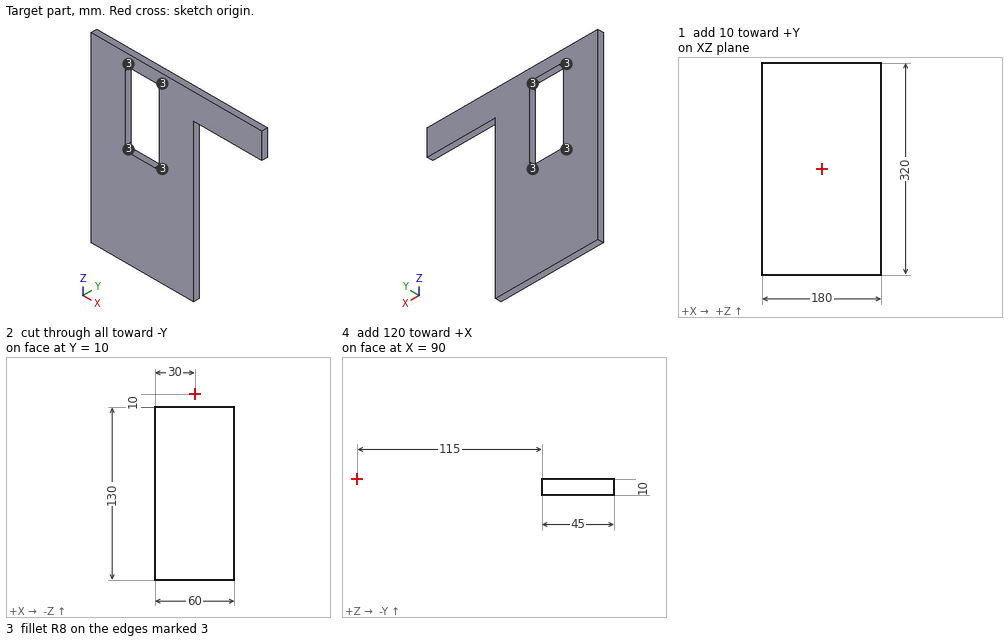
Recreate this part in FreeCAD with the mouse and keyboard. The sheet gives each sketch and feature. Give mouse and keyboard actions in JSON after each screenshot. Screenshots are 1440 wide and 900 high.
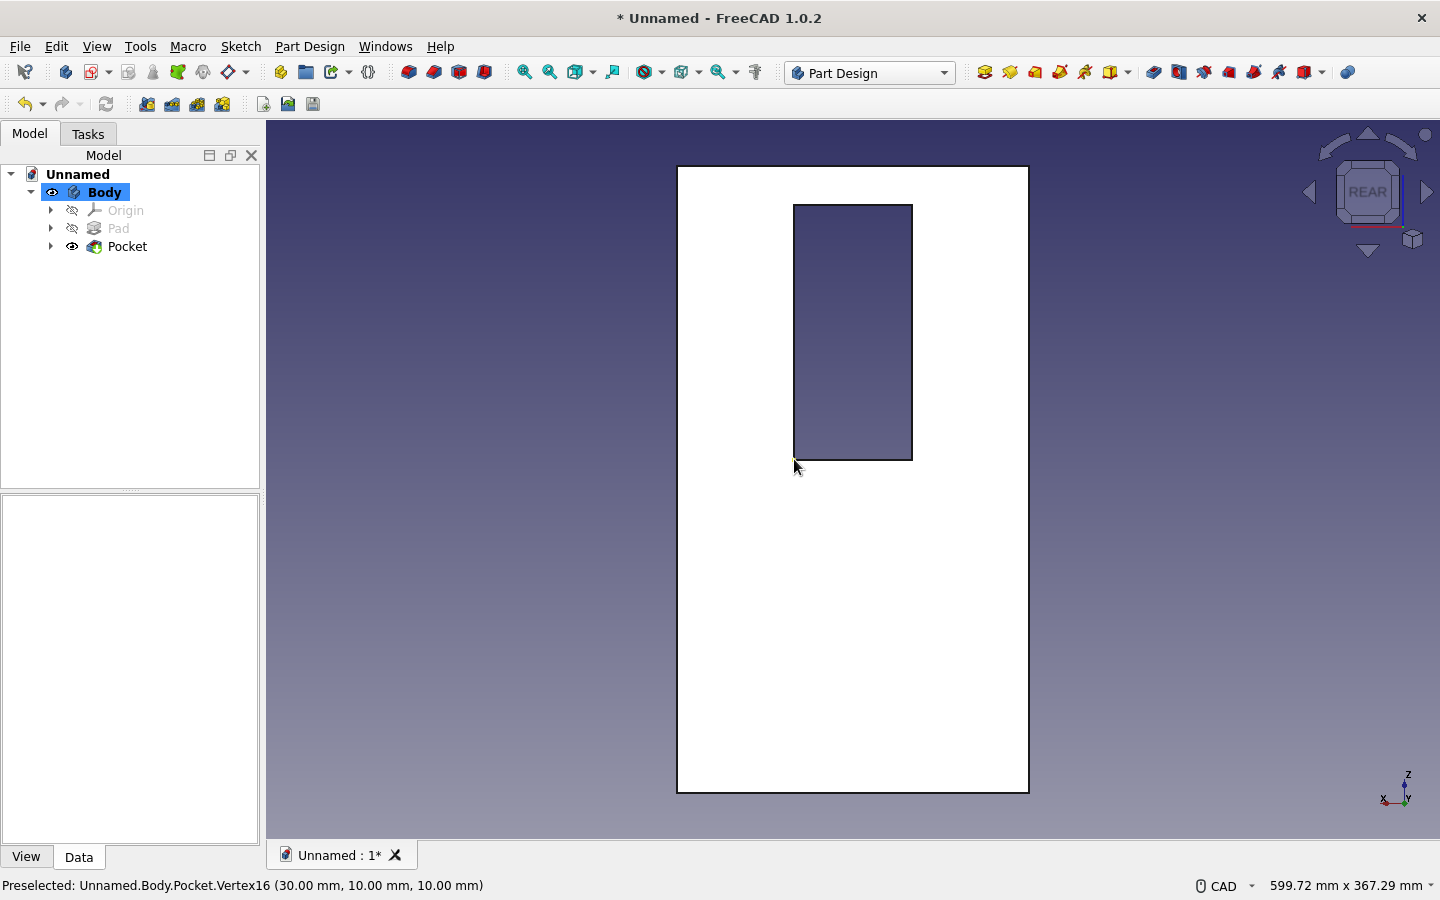
{"action": "key", "text": "0"}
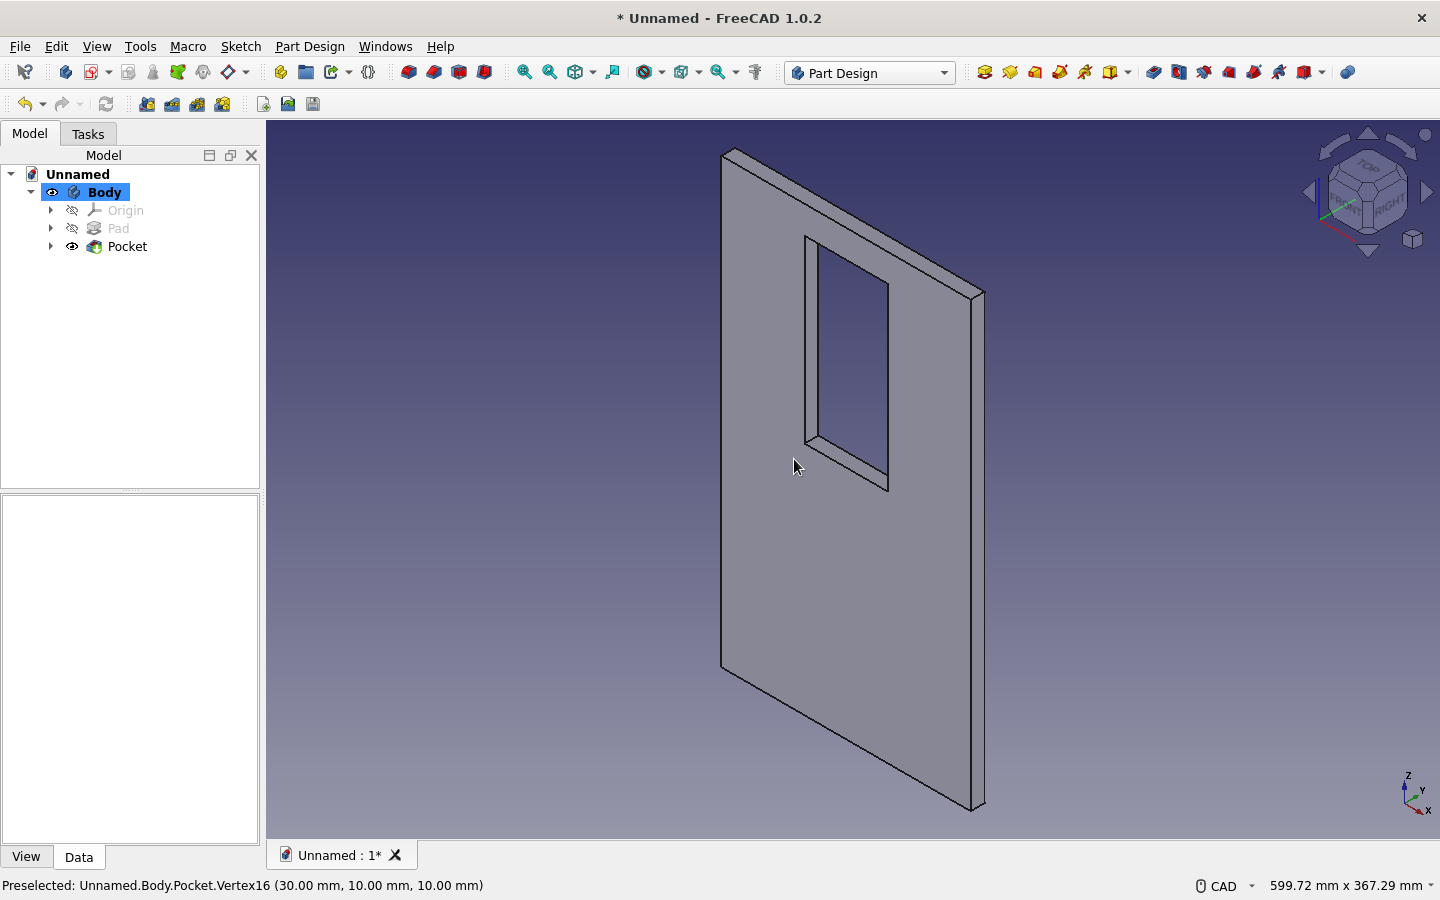
{"action": "scroll", "coordinate": [895, 486], "scroll_direction": "up", "scroll_amount": 4}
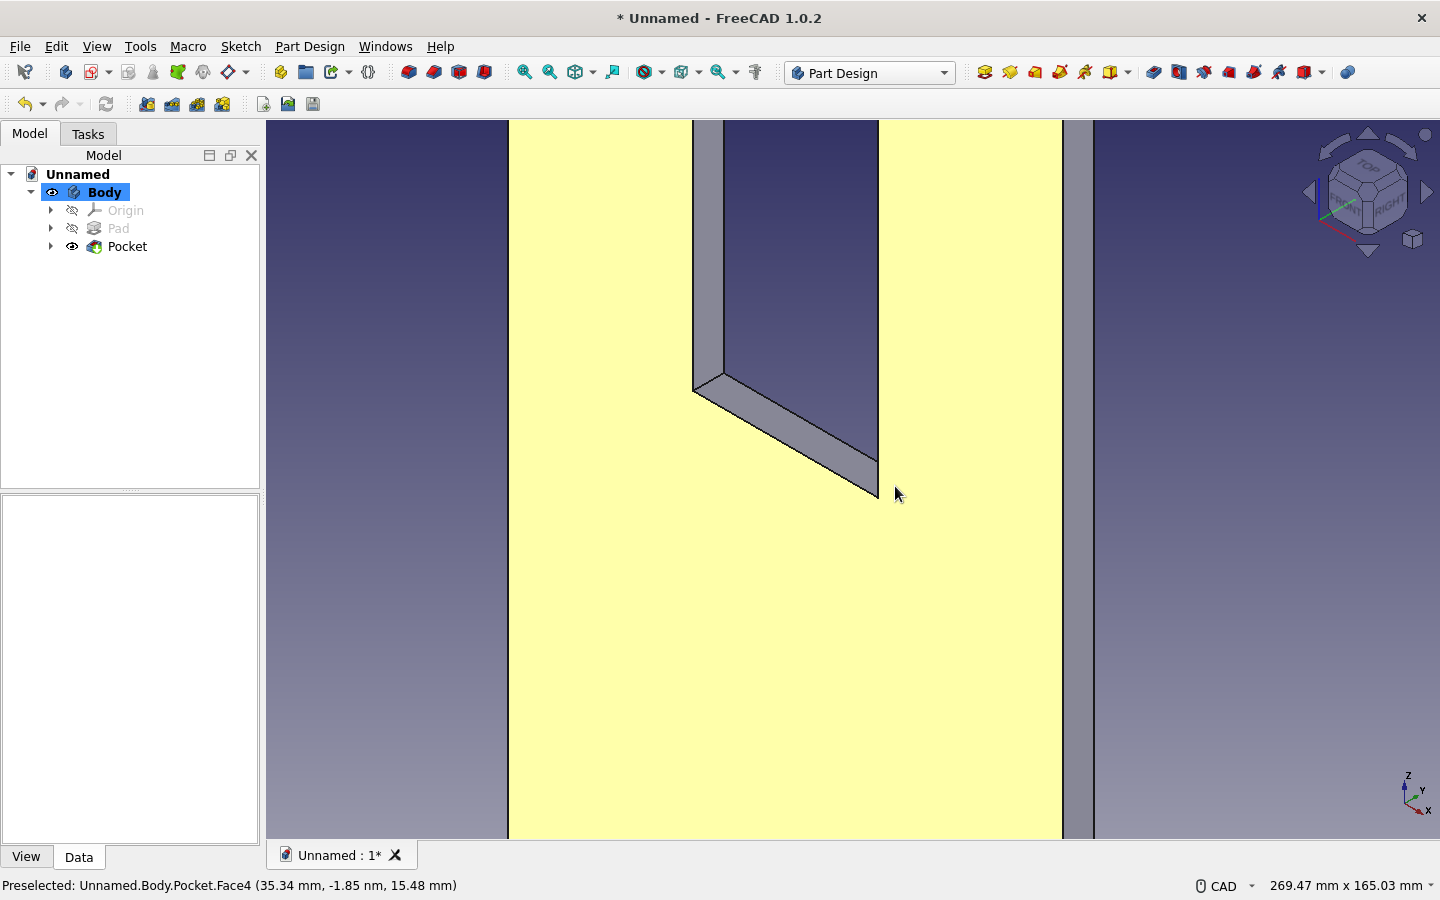
{"action": "key", "text": "v f"}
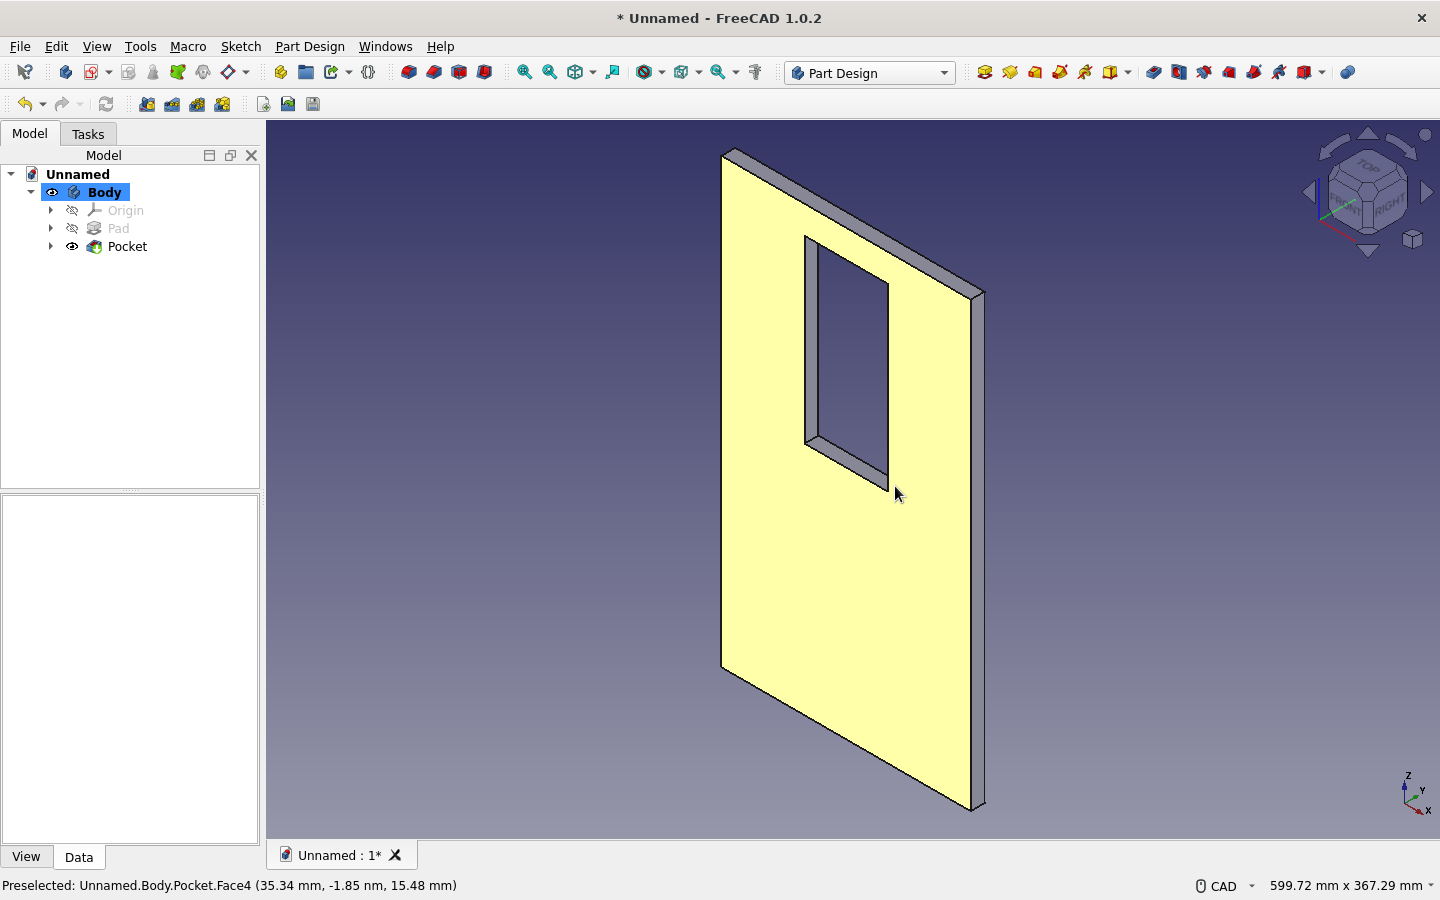
{"action": "key", "text": "2"}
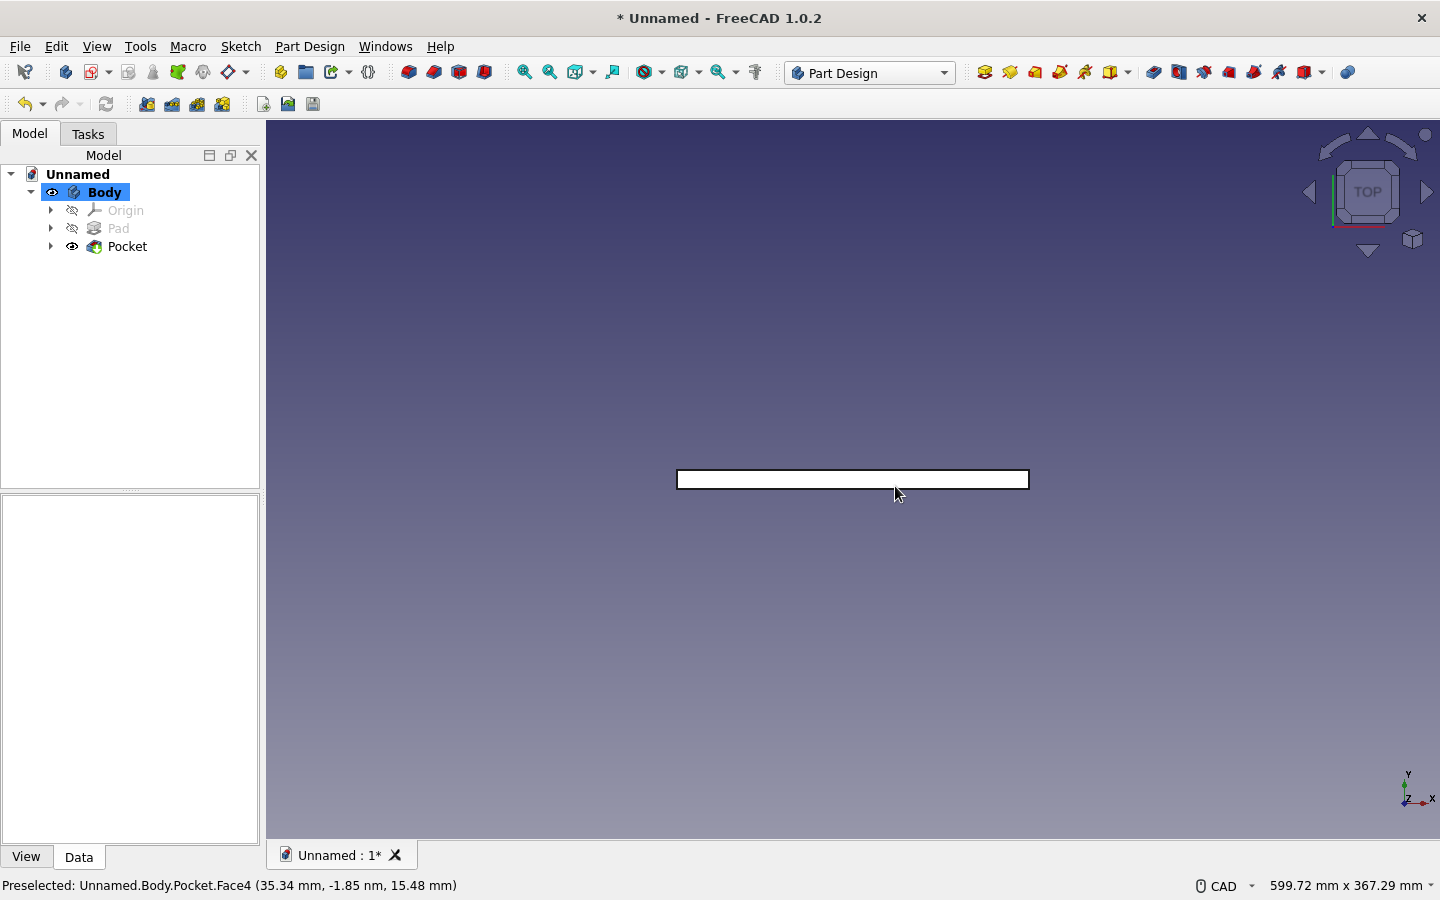
{"action": "key", "text": "v f"}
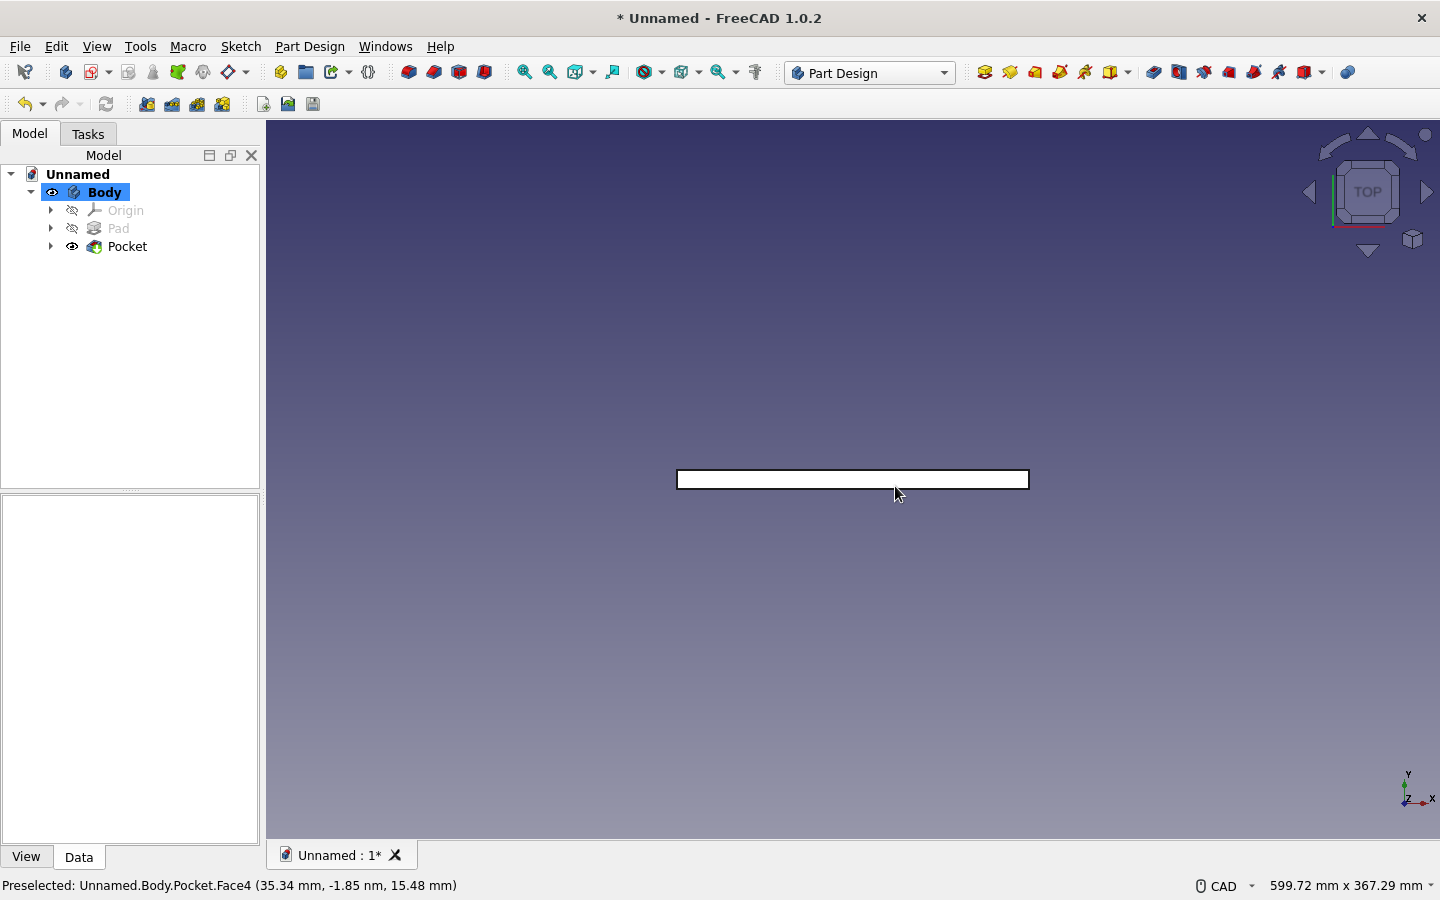
{"action": "scroll", "coordinate": [912, 478], "scroll_direction": "up", "scroll_amount": 4}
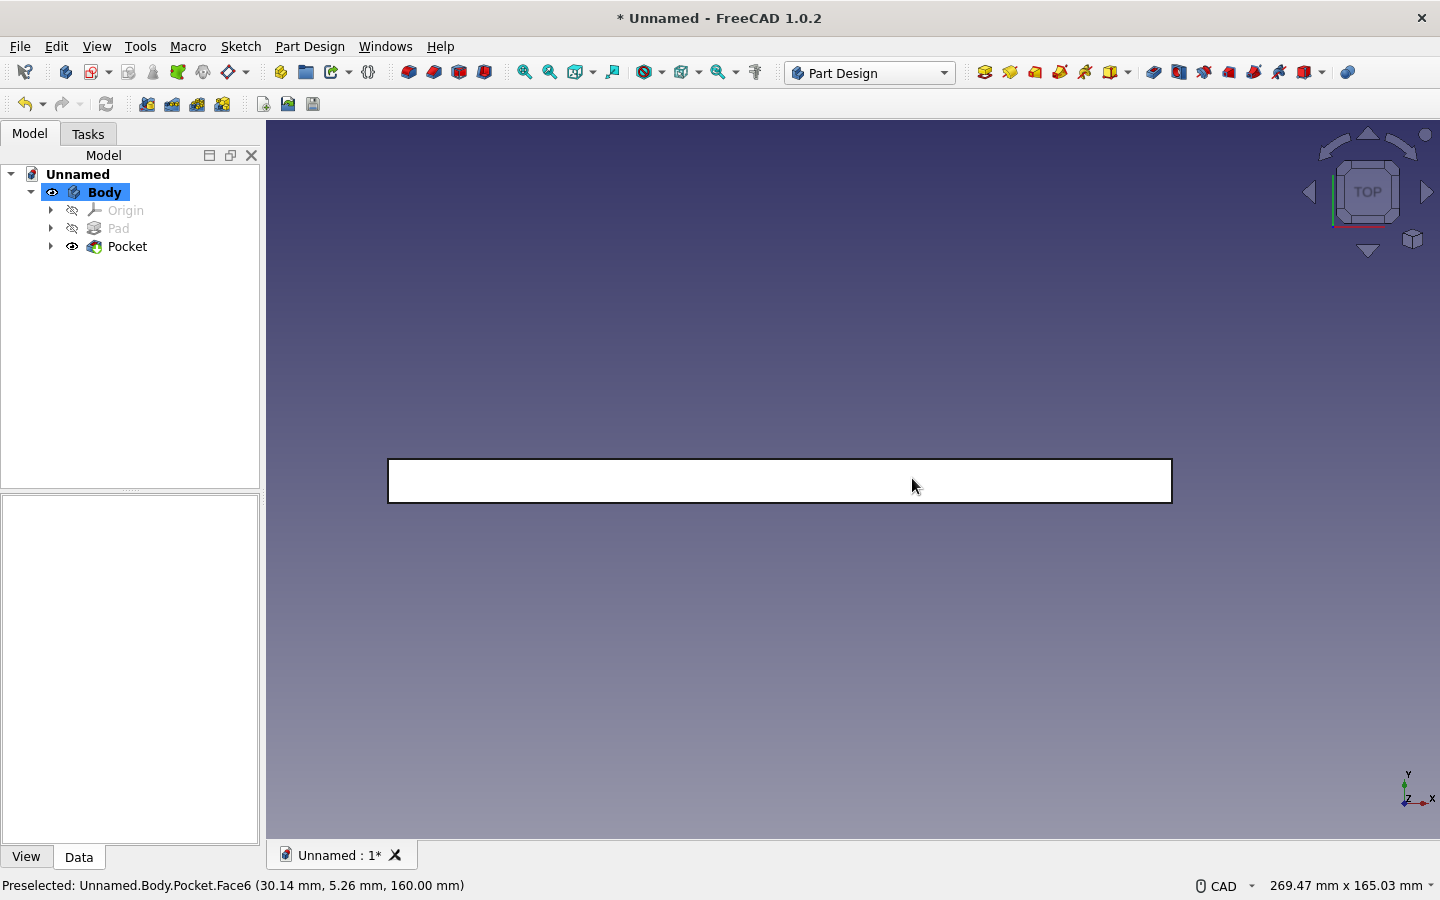
{"action": "left_click", "coordinate": [525, 72]}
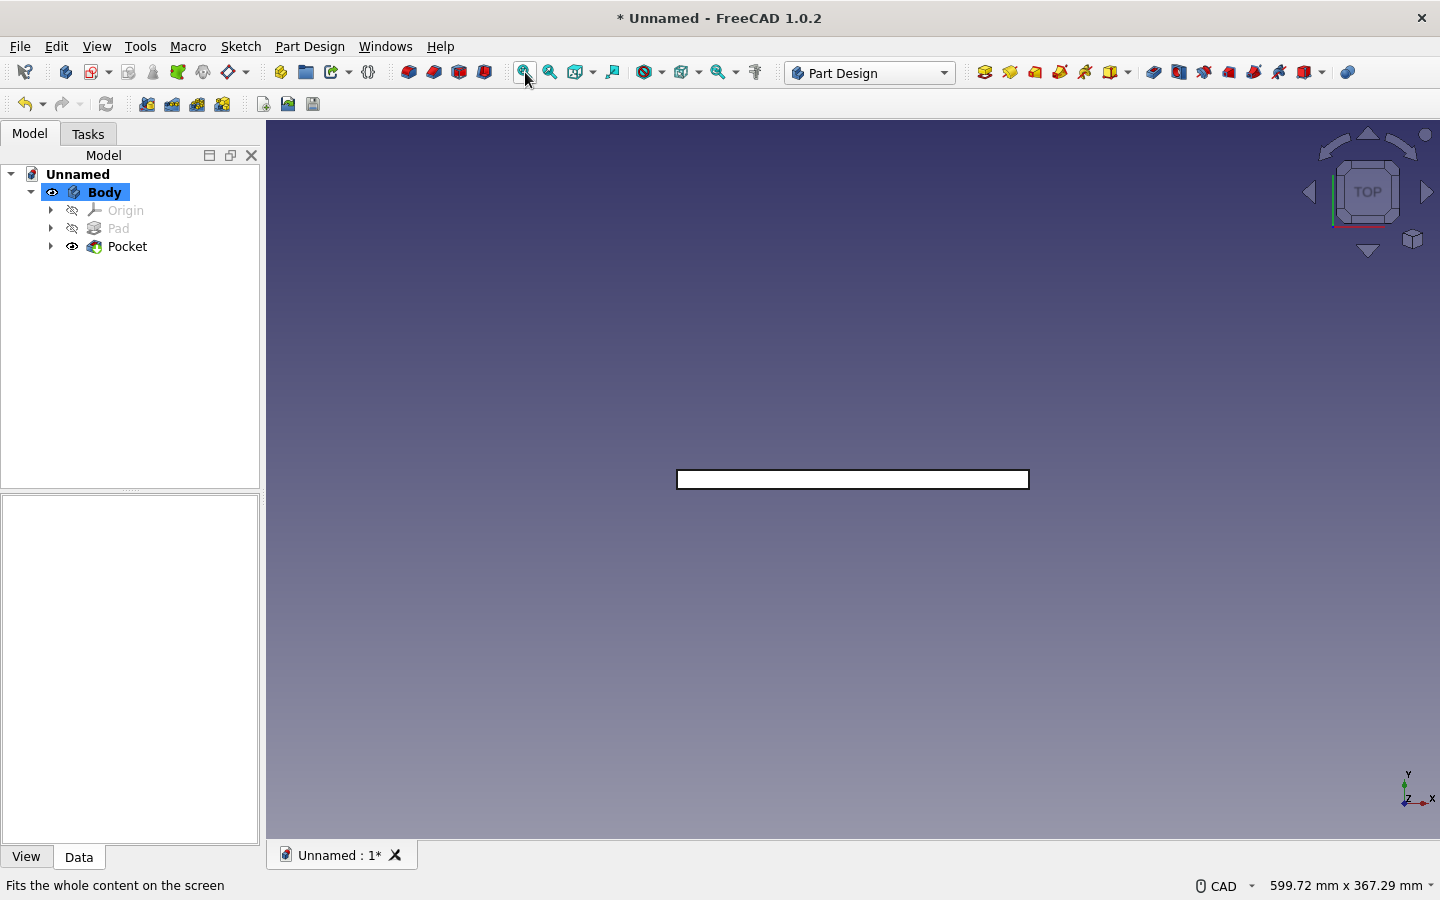
{"action": "key", "text": "1"}